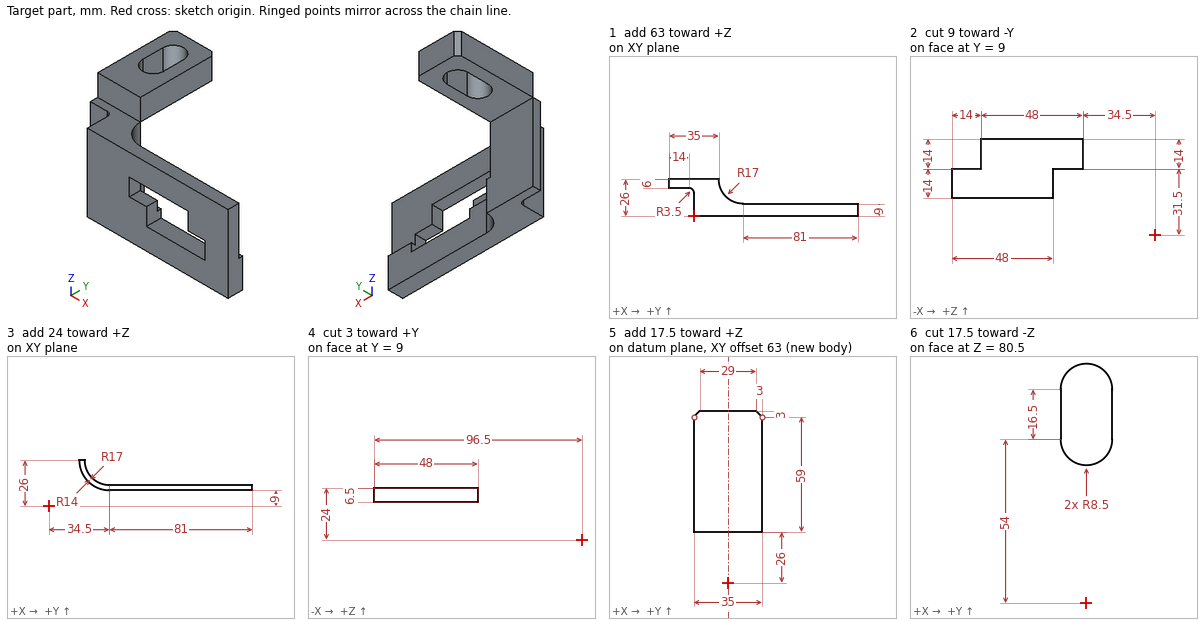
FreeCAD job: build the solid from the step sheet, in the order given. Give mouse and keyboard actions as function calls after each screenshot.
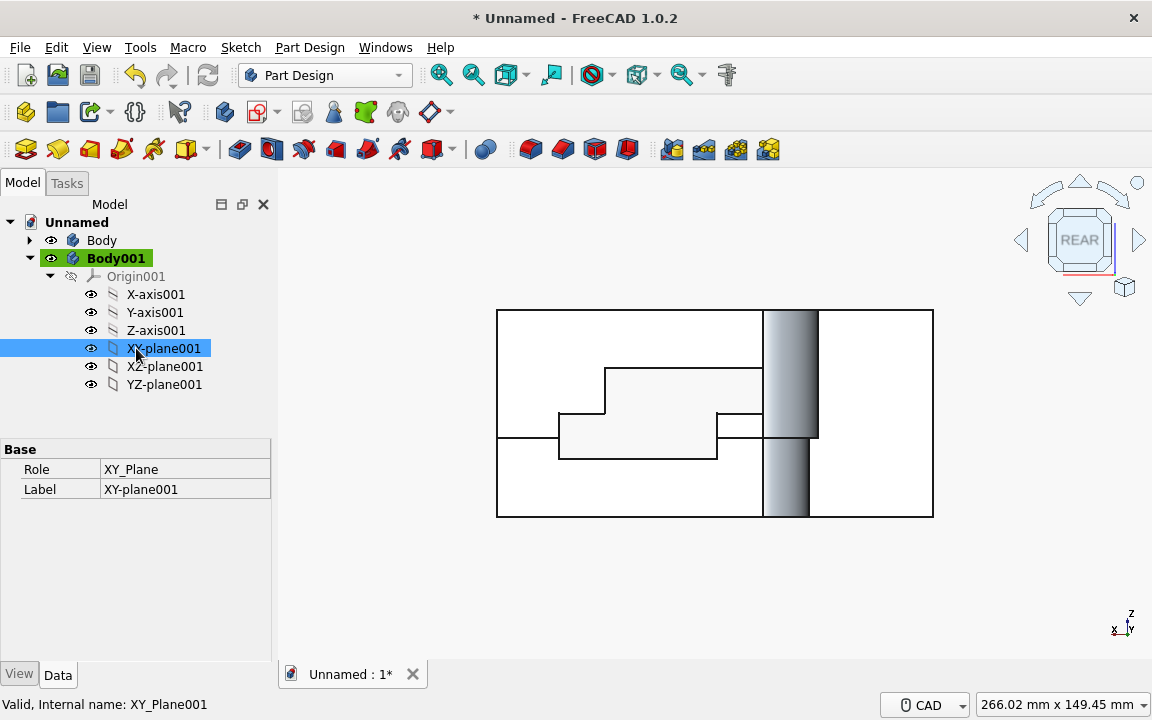
click(430, 112)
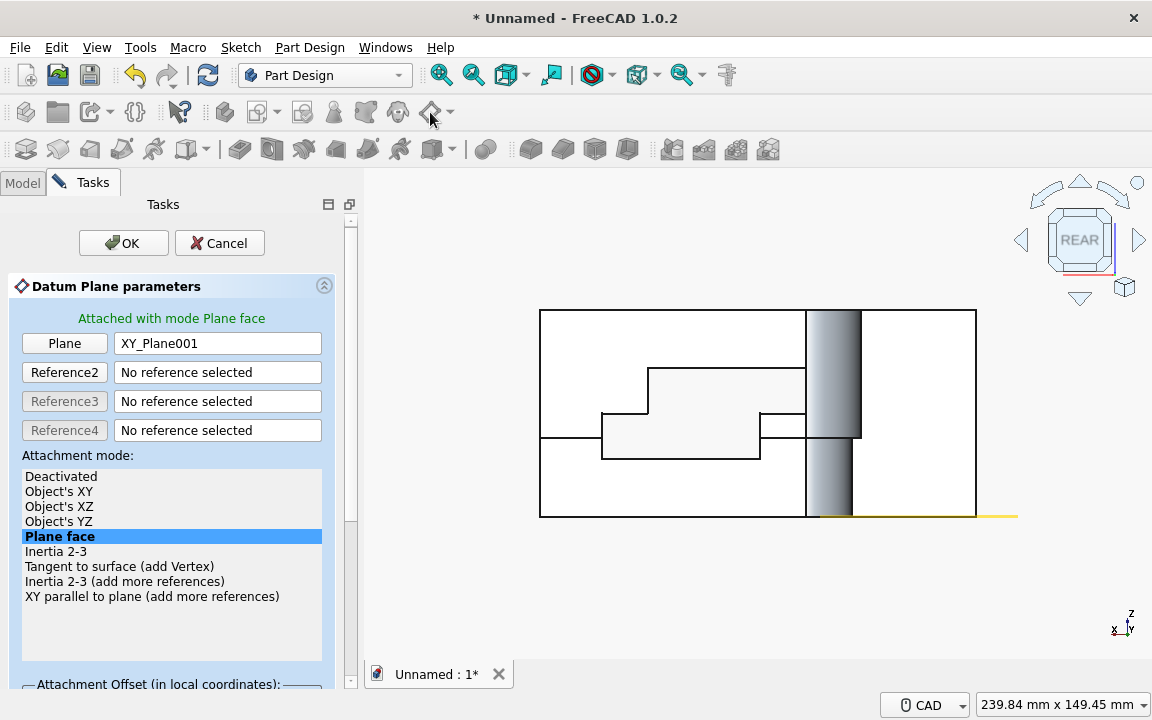
scroll(351, 451, down, 3)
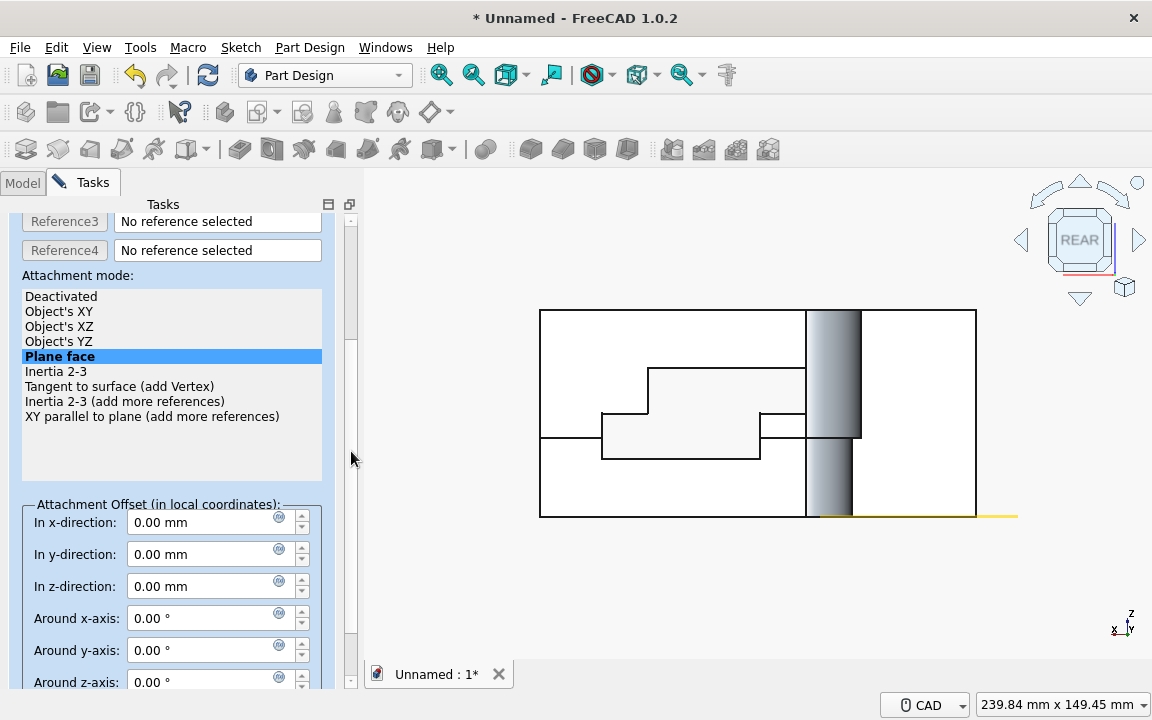
triple_click(210, 586)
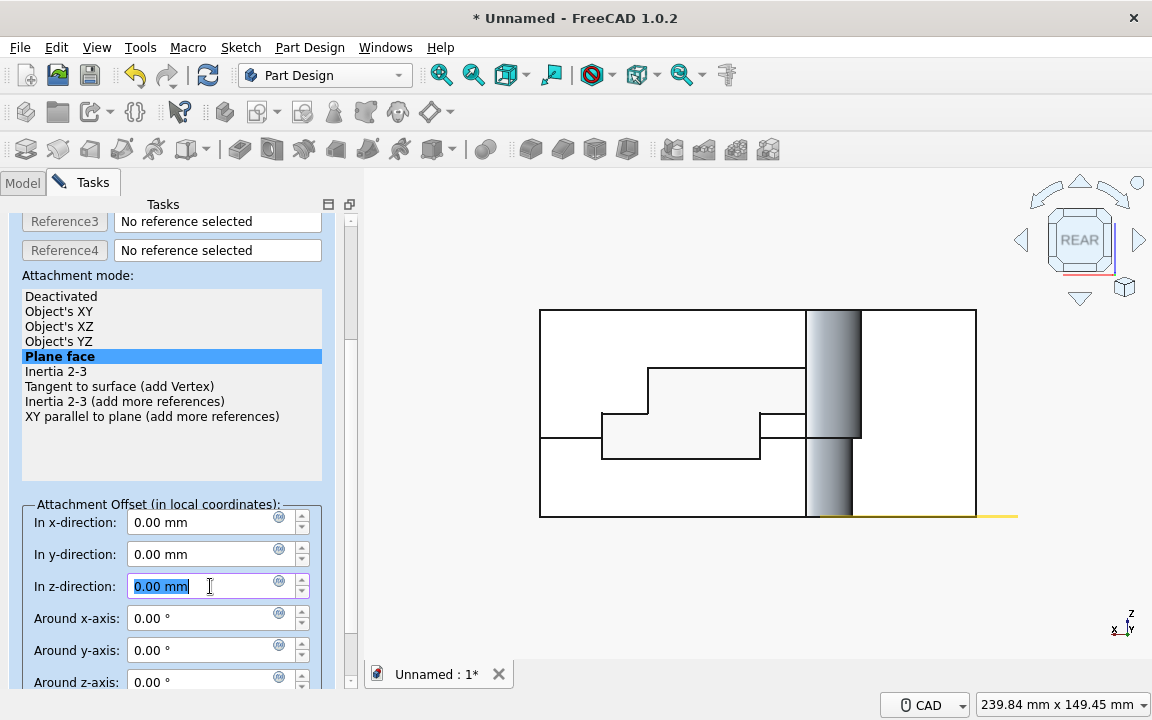
text(63)
key(Tab)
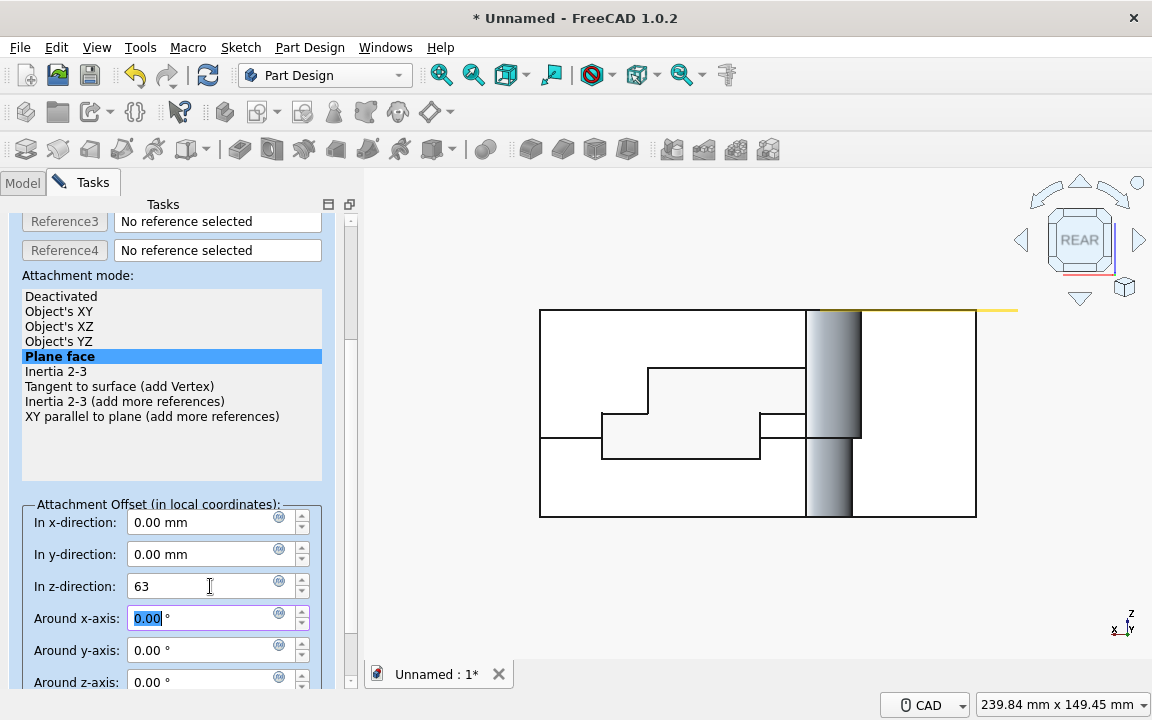
scroll(351, 451, up, 4)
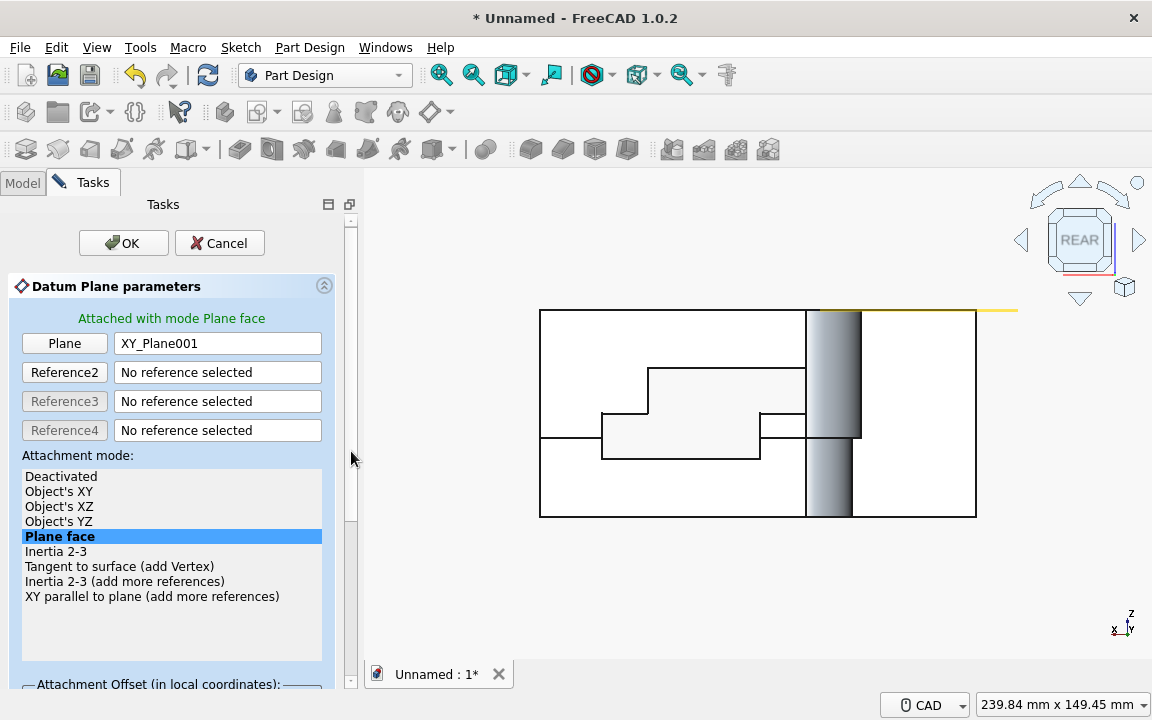
click(124, 243)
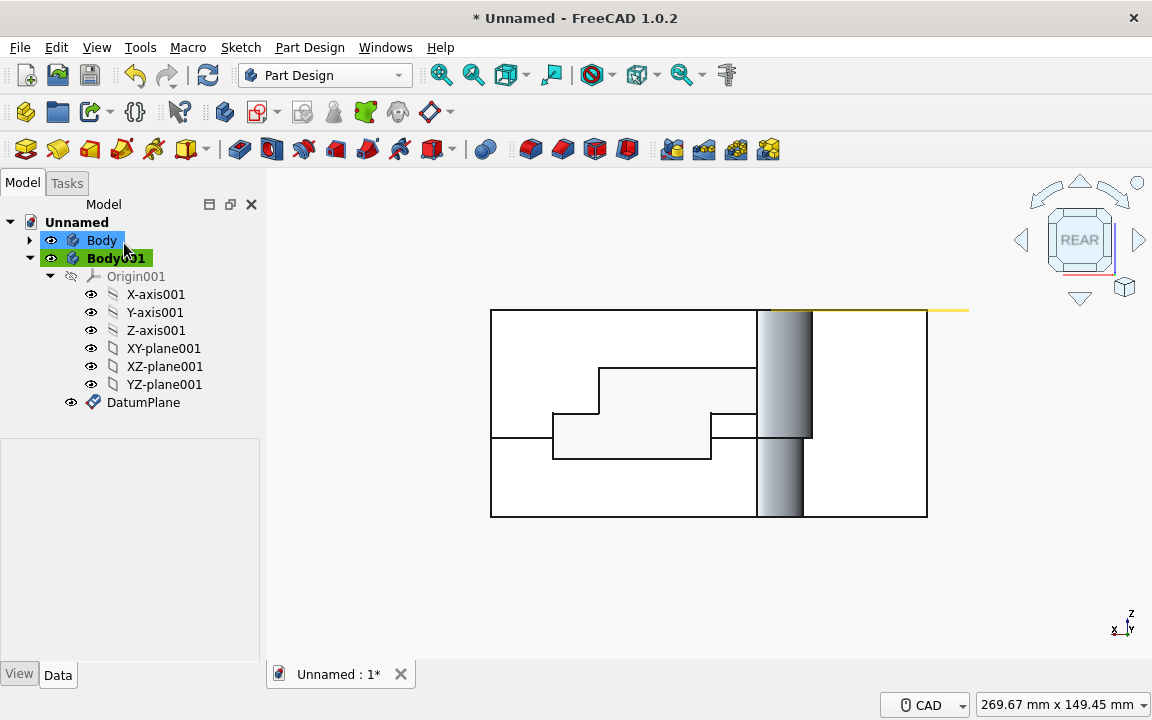
click(116, 402)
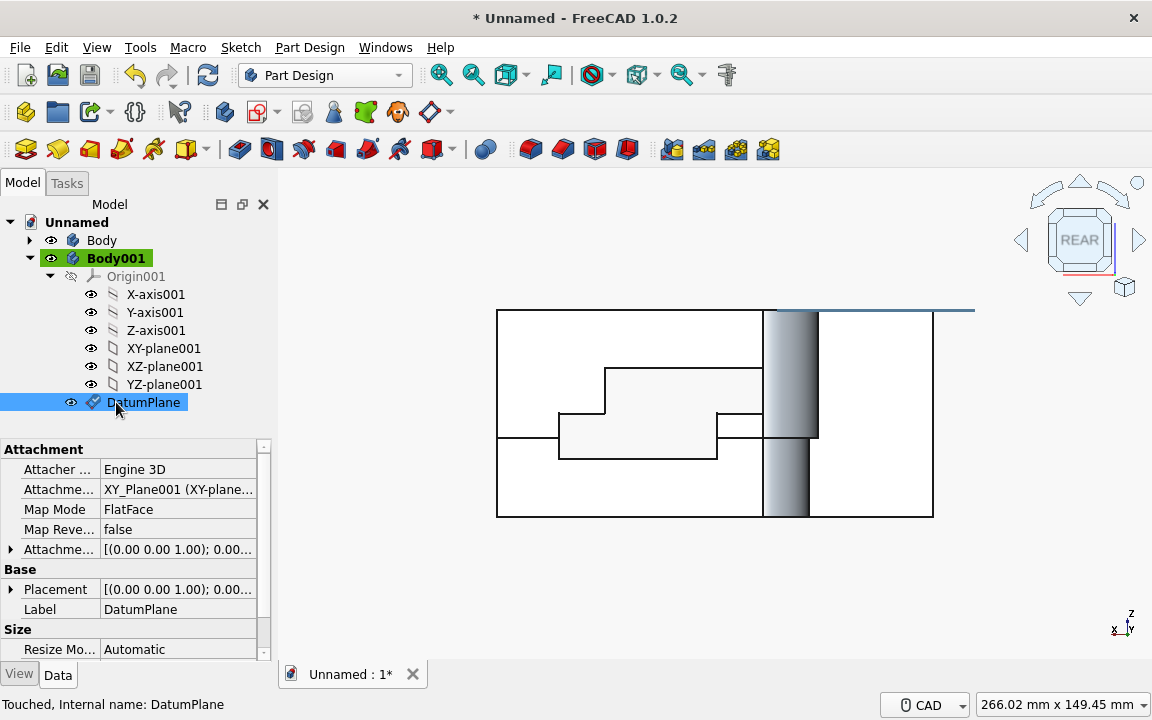
click(258, 112)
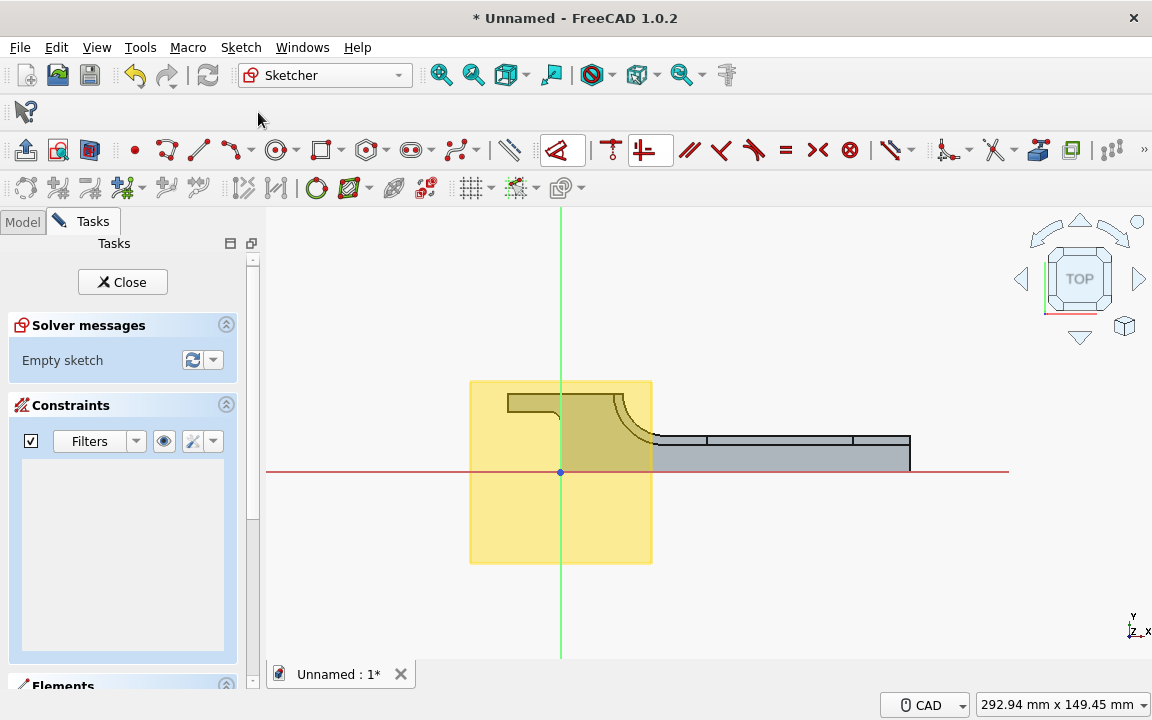
scroll(987, 631, down, 1)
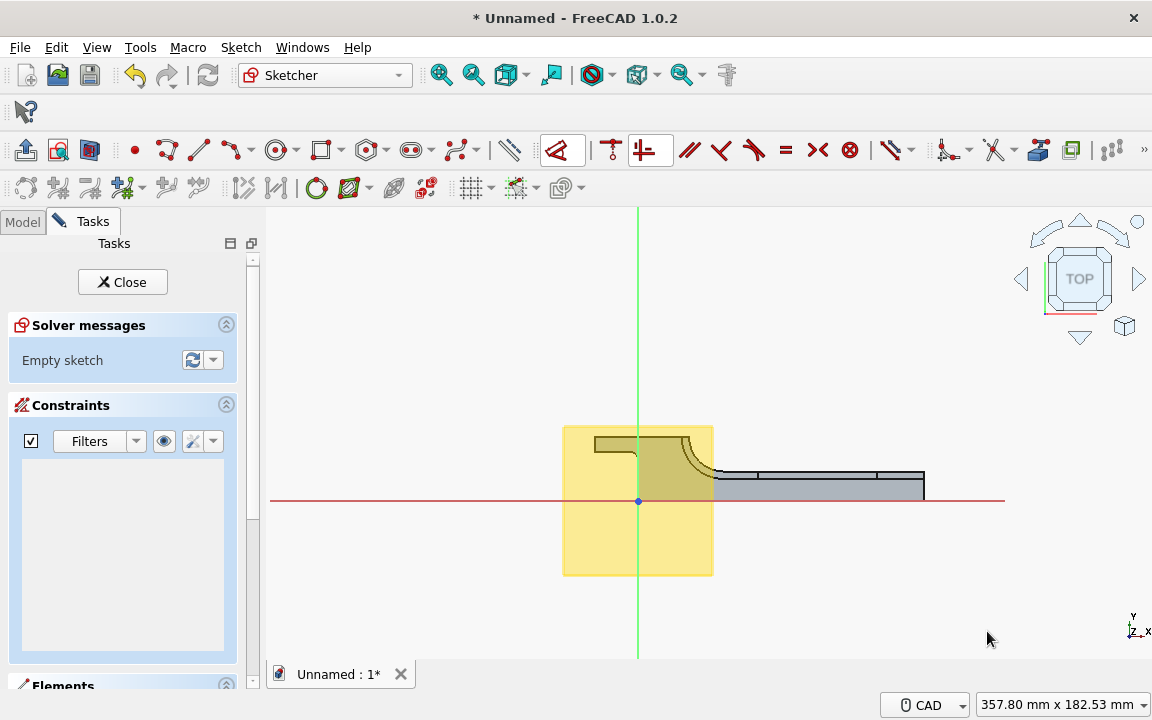
key(g)
key(m)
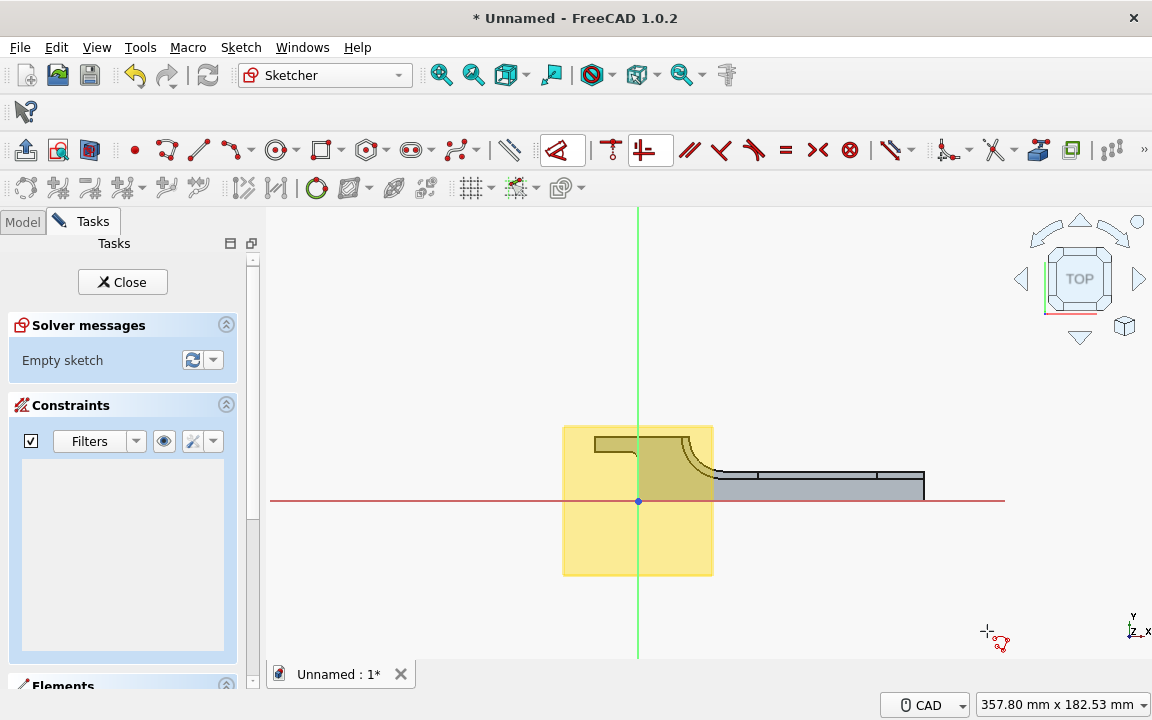
click(682, 437)
click(682, 291)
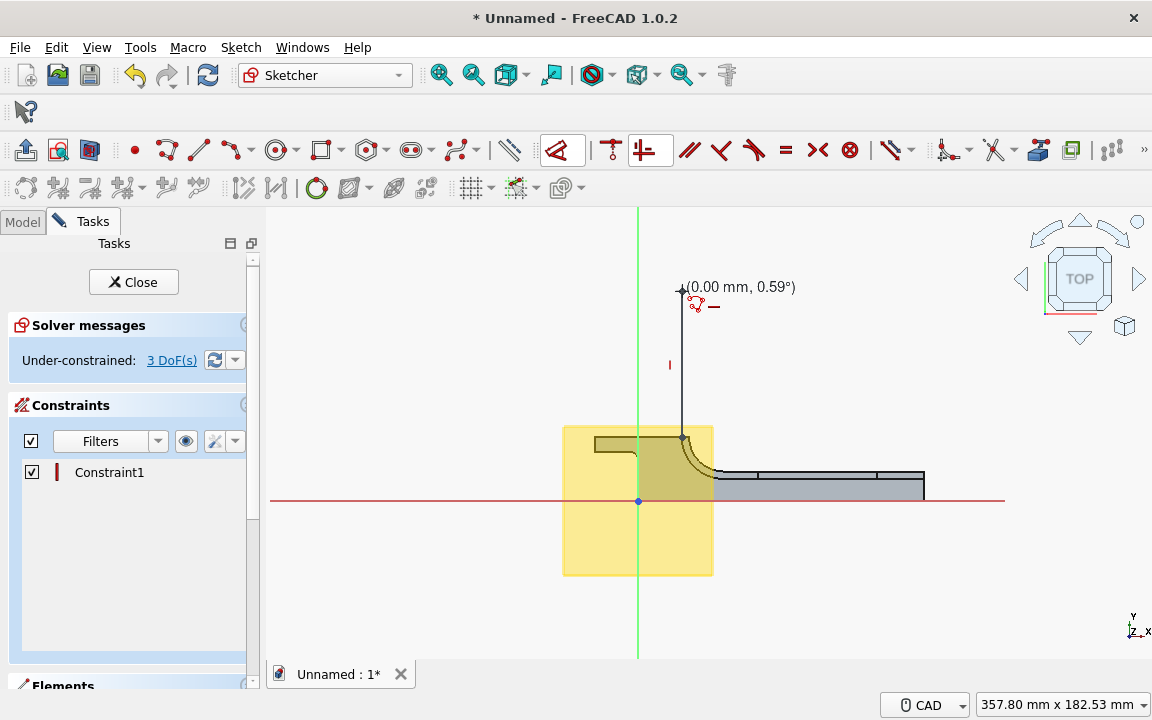
scroll(674, 283, up, 3)